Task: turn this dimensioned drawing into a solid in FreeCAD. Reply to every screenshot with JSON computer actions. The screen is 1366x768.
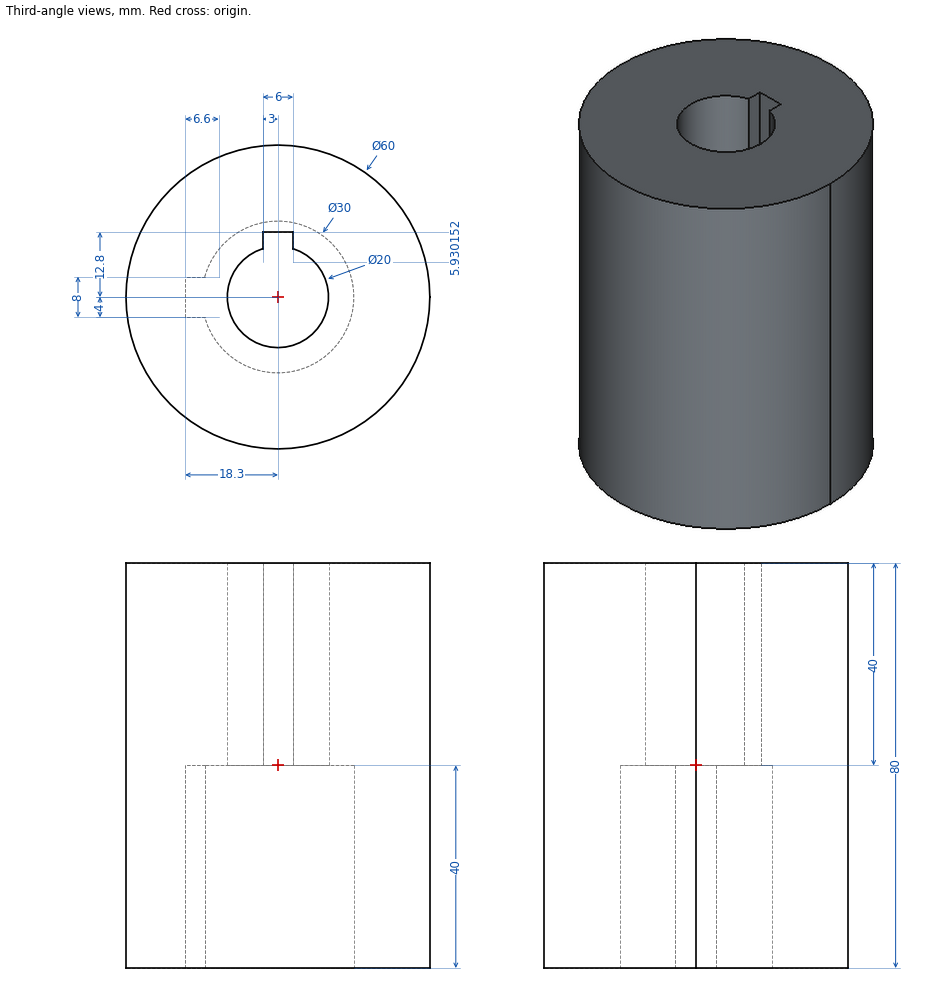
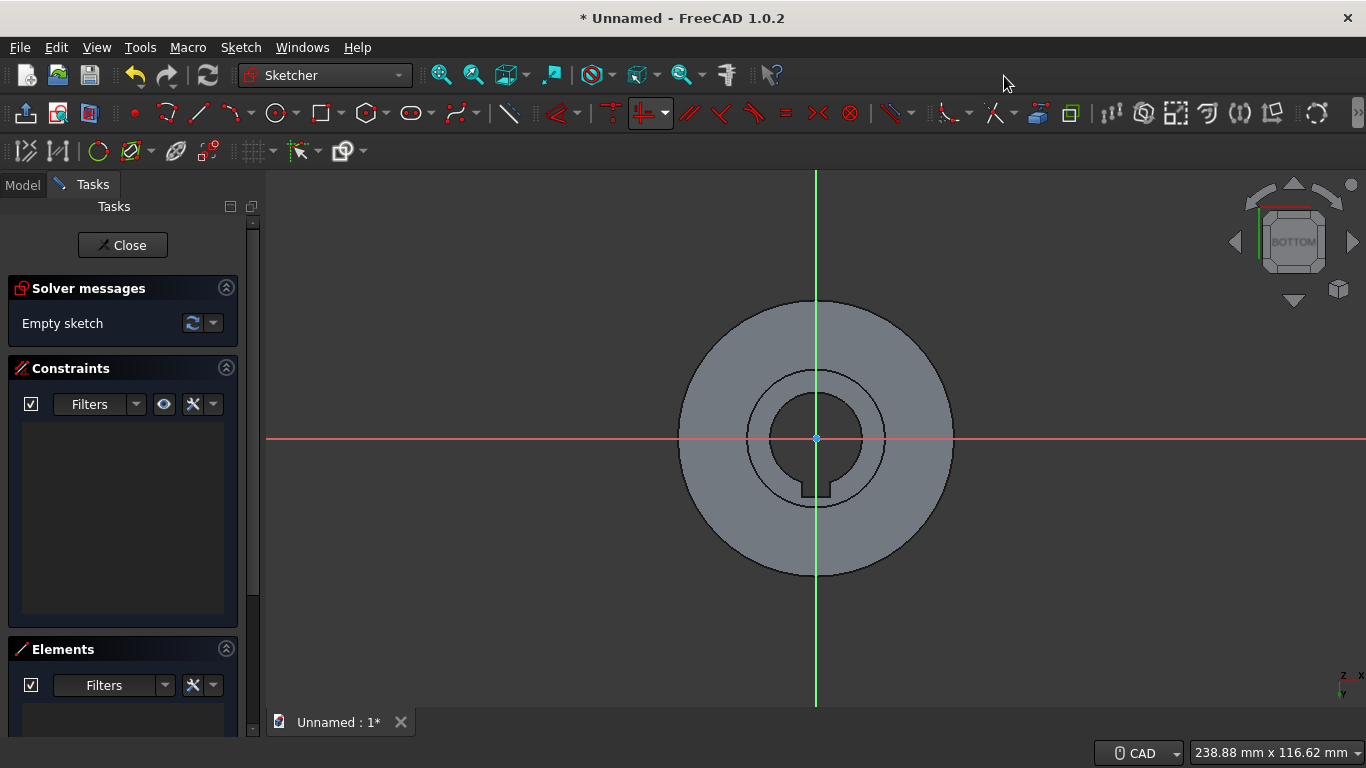
{"action": "scroll", "coordinate": [778, 439], "scroll_direction": "up", "scroll_amount": 10}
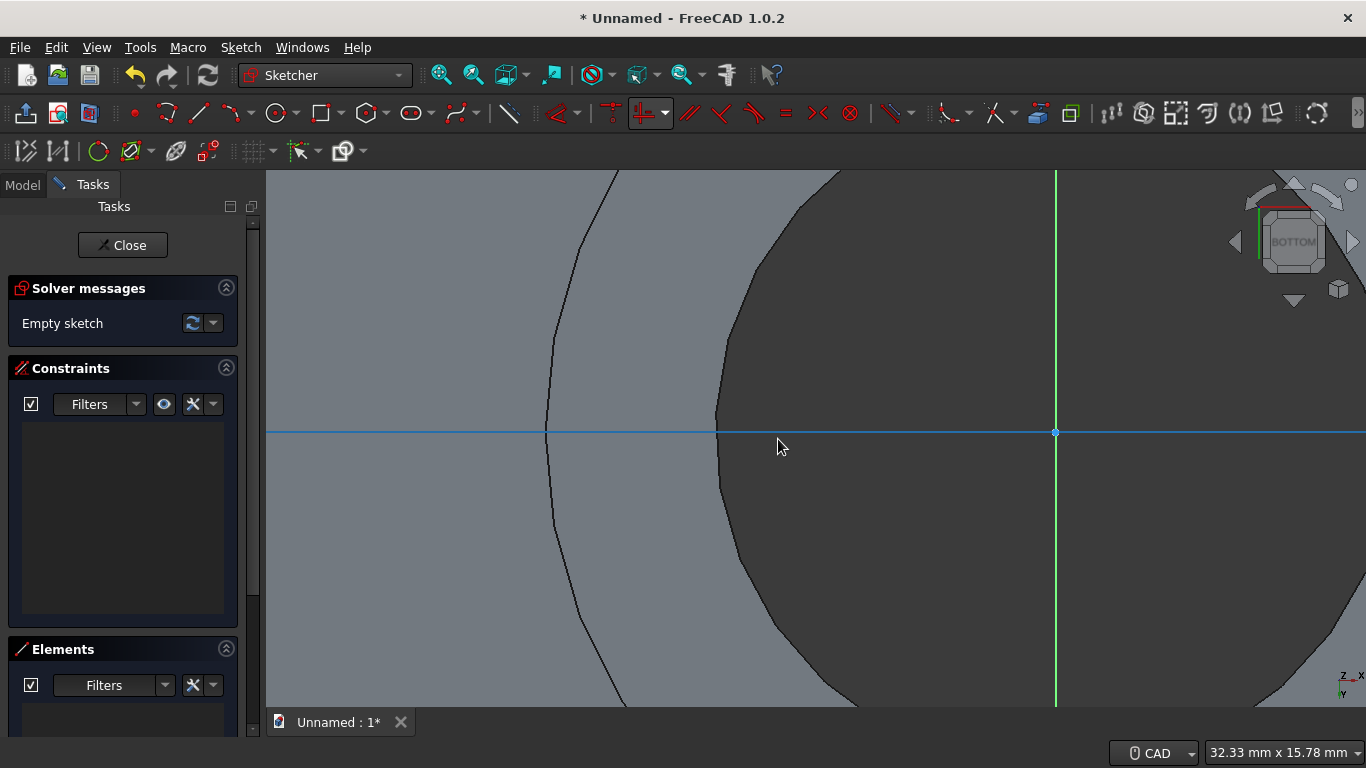
{"action": "key", "text": "g r"}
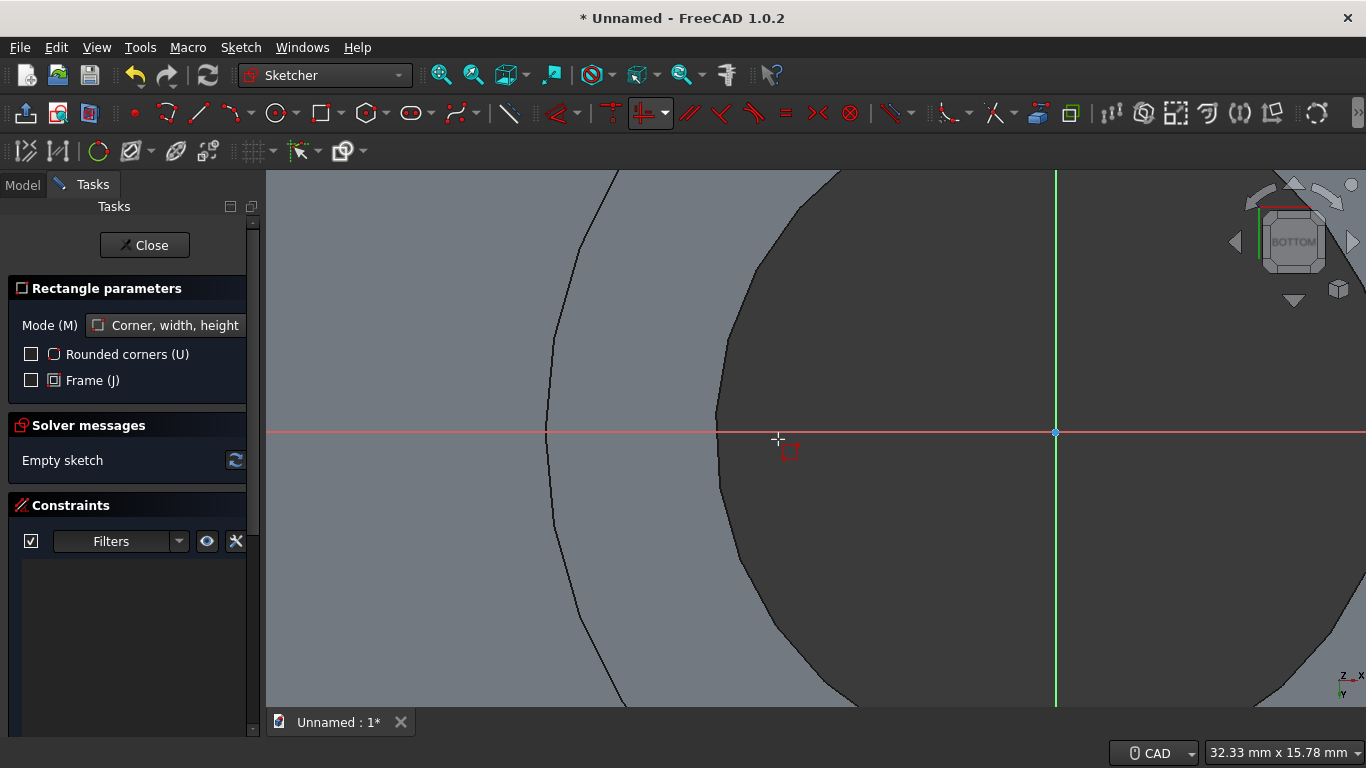
{"action": "left_click", "coordinate": [433, 296]}
{"action": "mouse_move", "coordinate": [658, 568]}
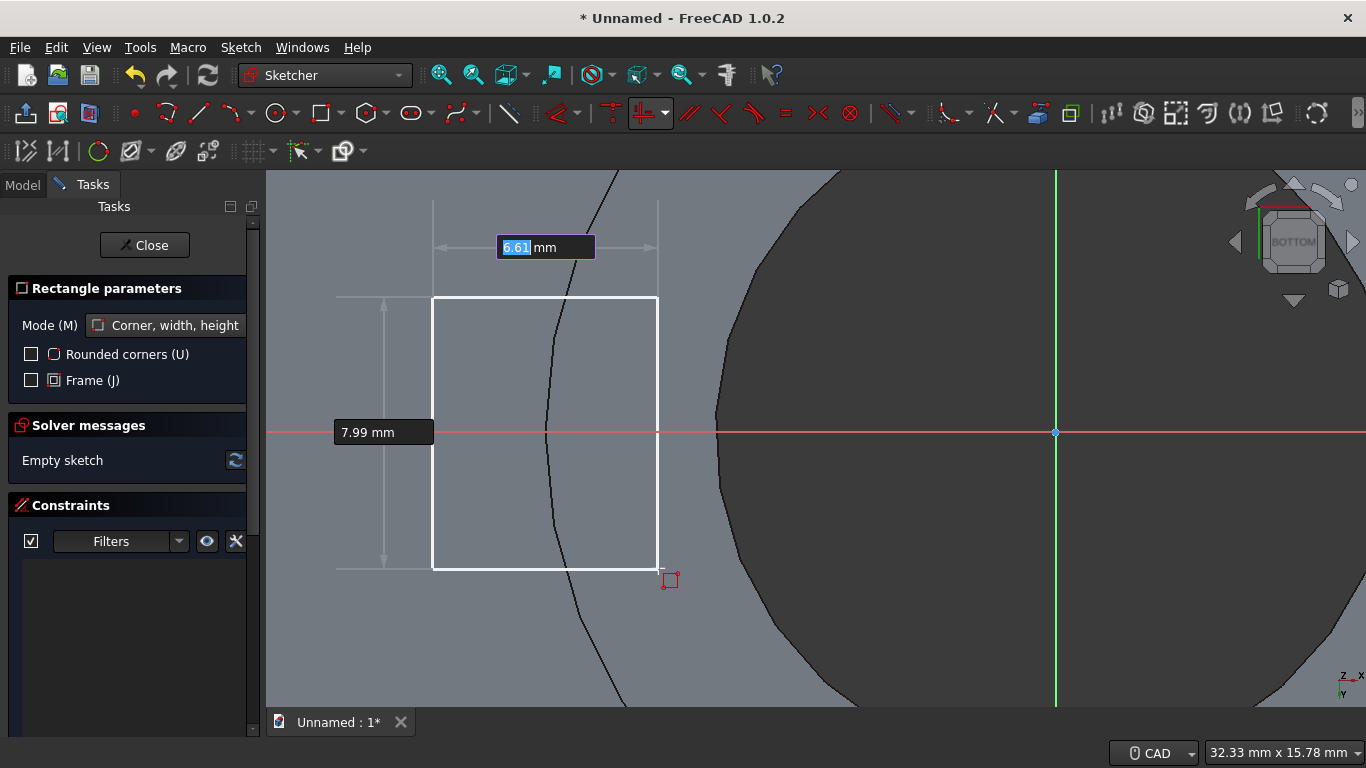
{"action": "type", "text": "6.6"}
{"action": "key", "text": "Tab"}
{"action": "type", "text": "8"}
{"action": "key", "text": "Return"}
{"action": "key", "text": "Escape"}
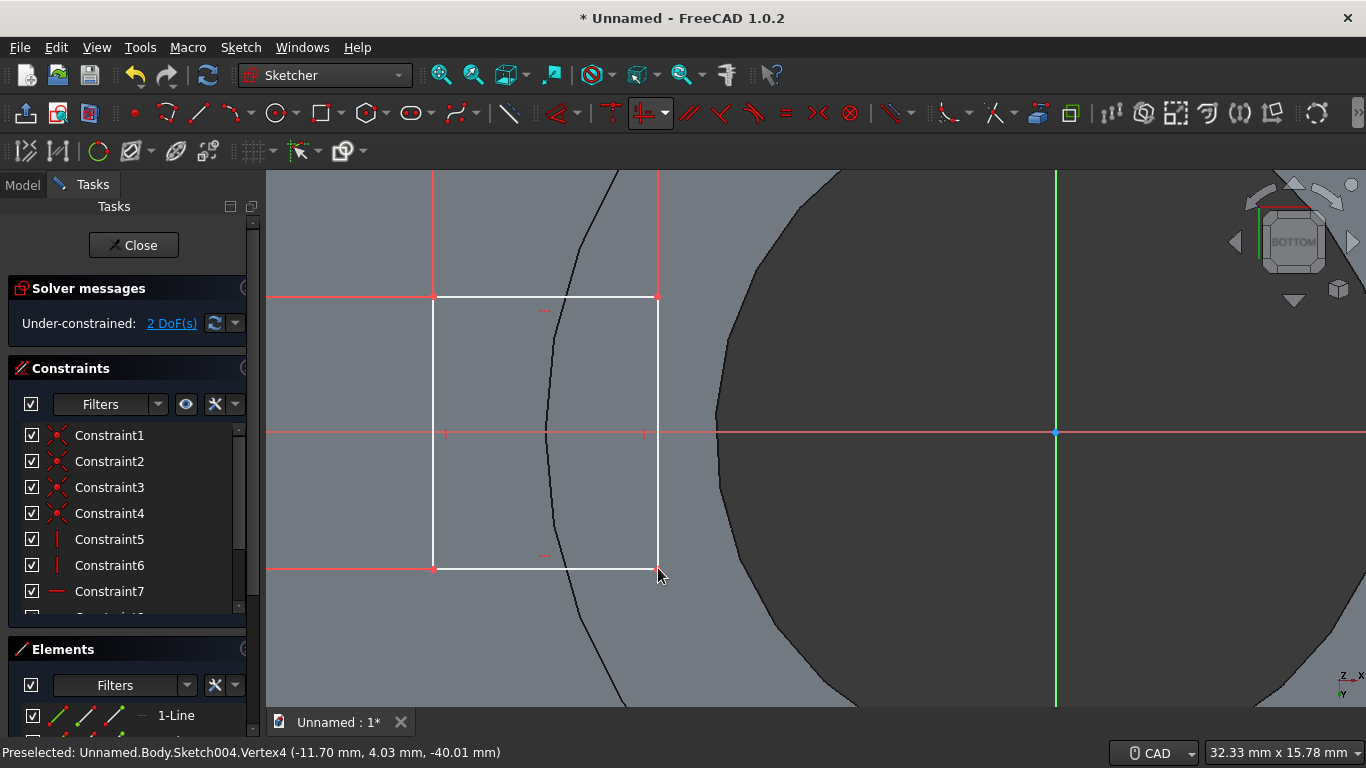
{"action": "left_click", "coordinate": [556, 114]}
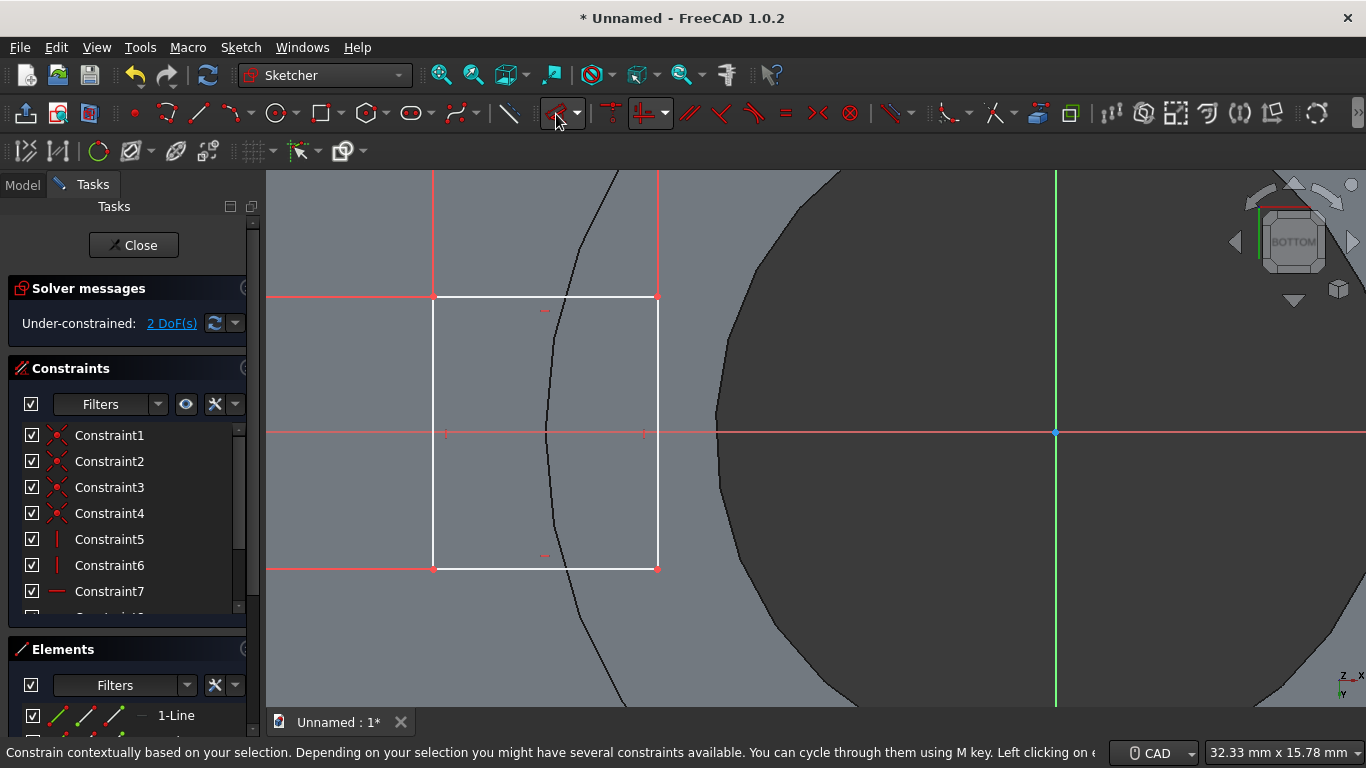
{"action": "left_click", "coordinate": [433, 297]}
{"action": "left_click", "coordinate": [399, 365]}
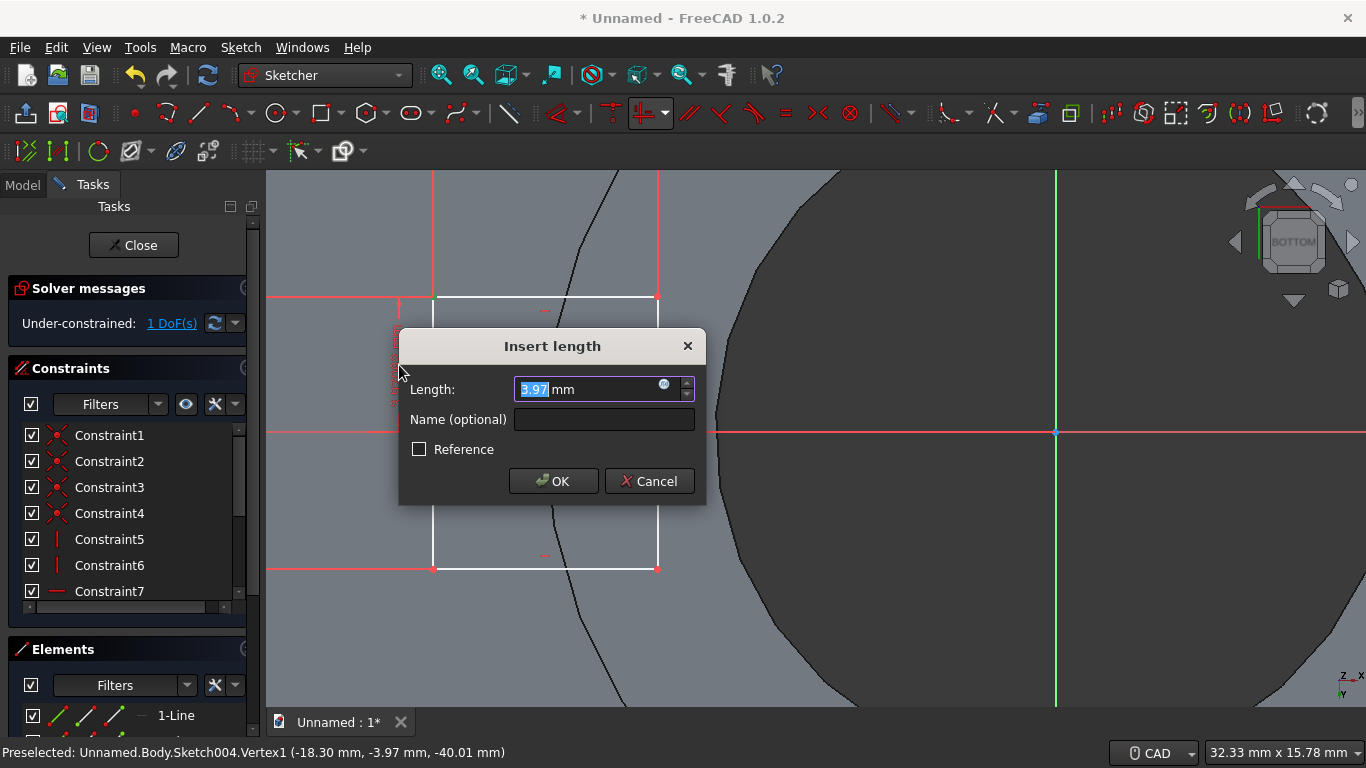
{"action": "type", "text": "4"}
{"action": "key", "text": "Return"}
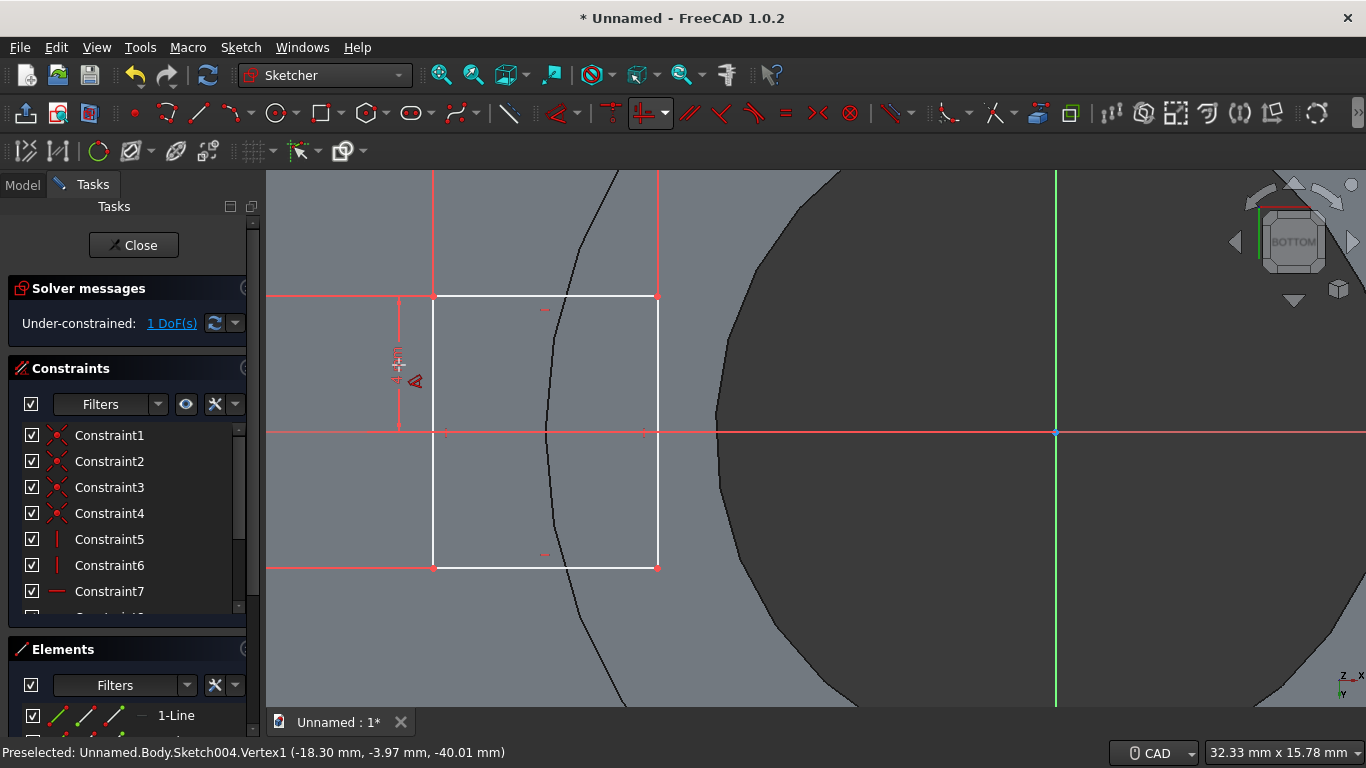
{"action": "left_click", "coordinate": [433, 296]}
{"action": "left_click", "coordinate": [744, 262]}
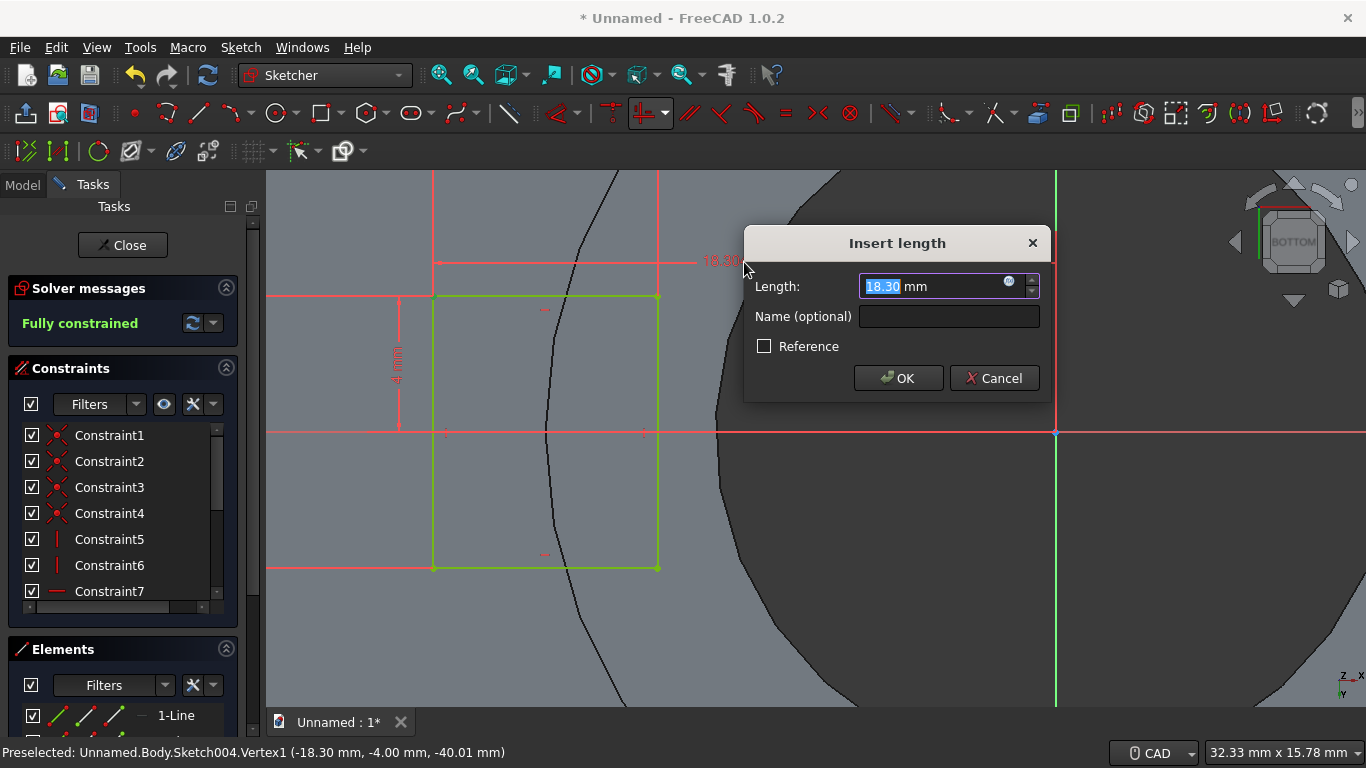
{"action": "type", "text": "18.3"}
{"action": "key", "text": "Return"}
{"action": "key", "text": "Escape"}